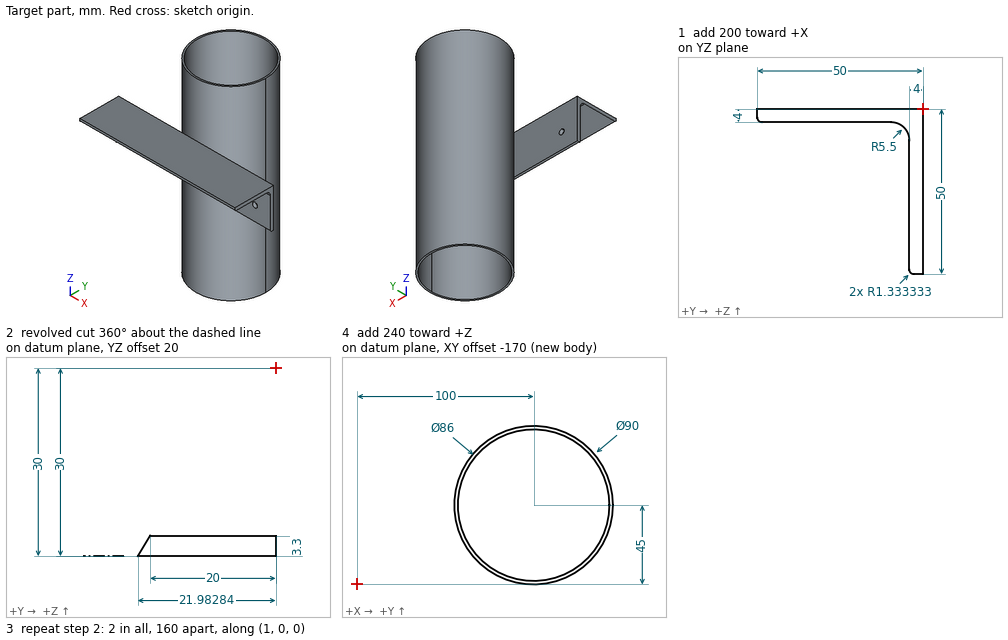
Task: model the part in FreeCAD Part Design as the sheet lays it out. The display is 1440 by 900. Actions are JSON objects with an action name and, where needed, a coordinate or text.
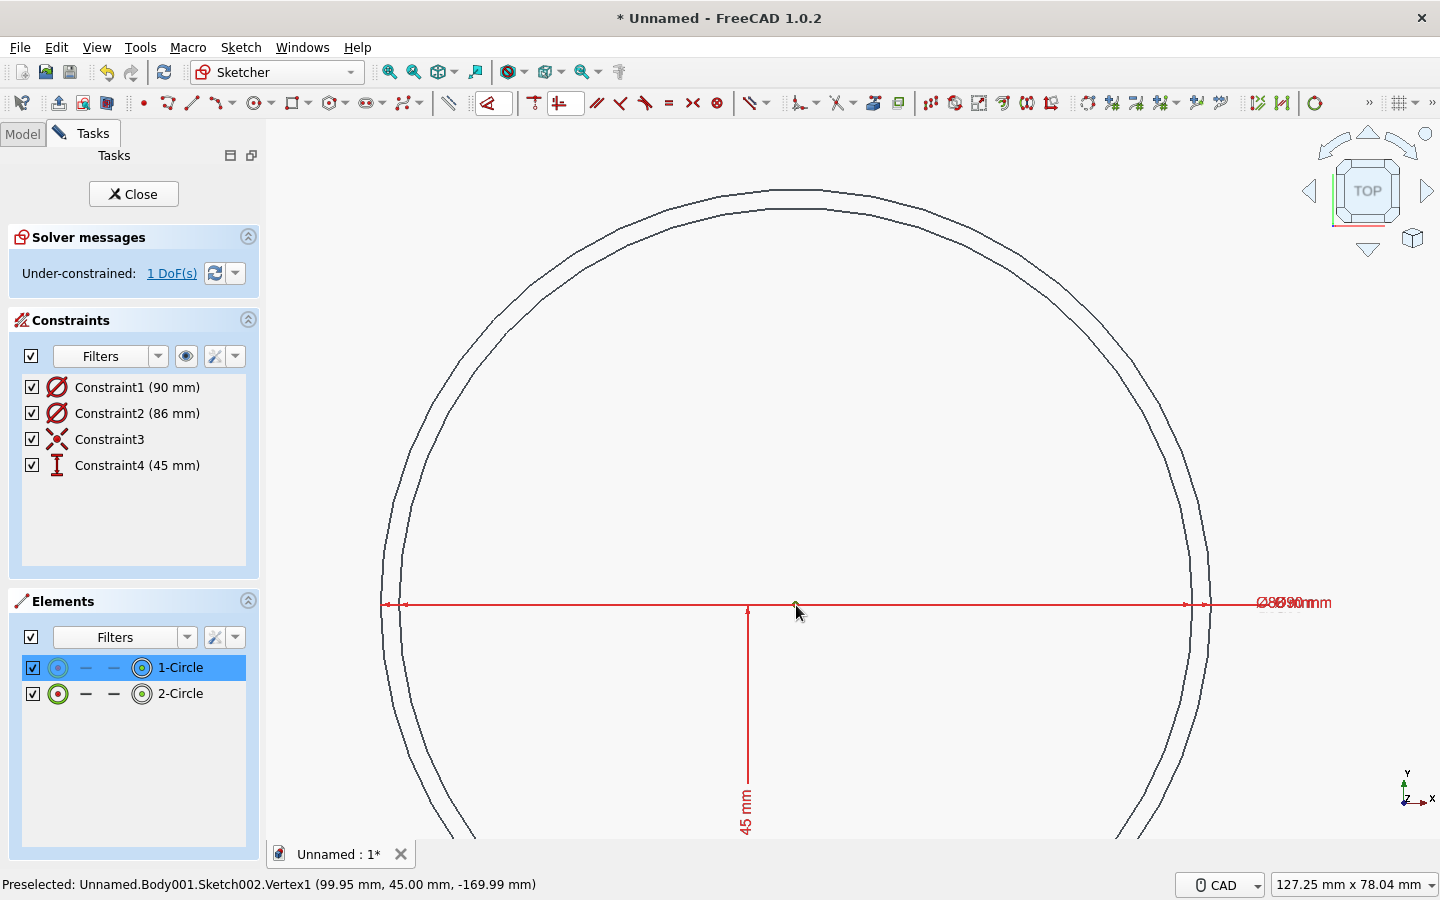
{"action": "left_click", "coordinate": [506, 104]}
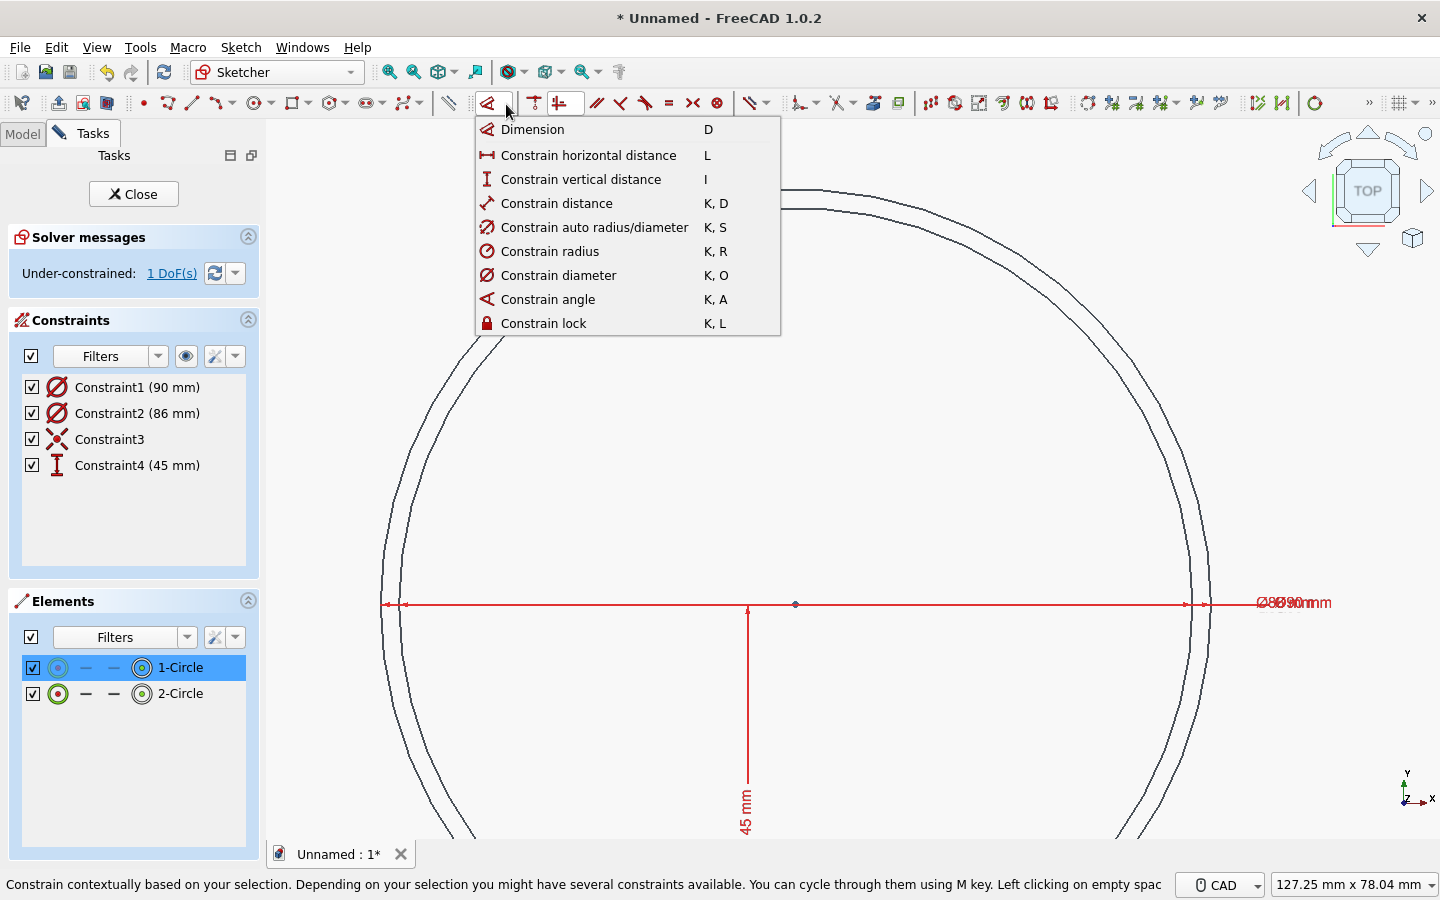
{"action": "left_click", "coordinate": [628, 155]}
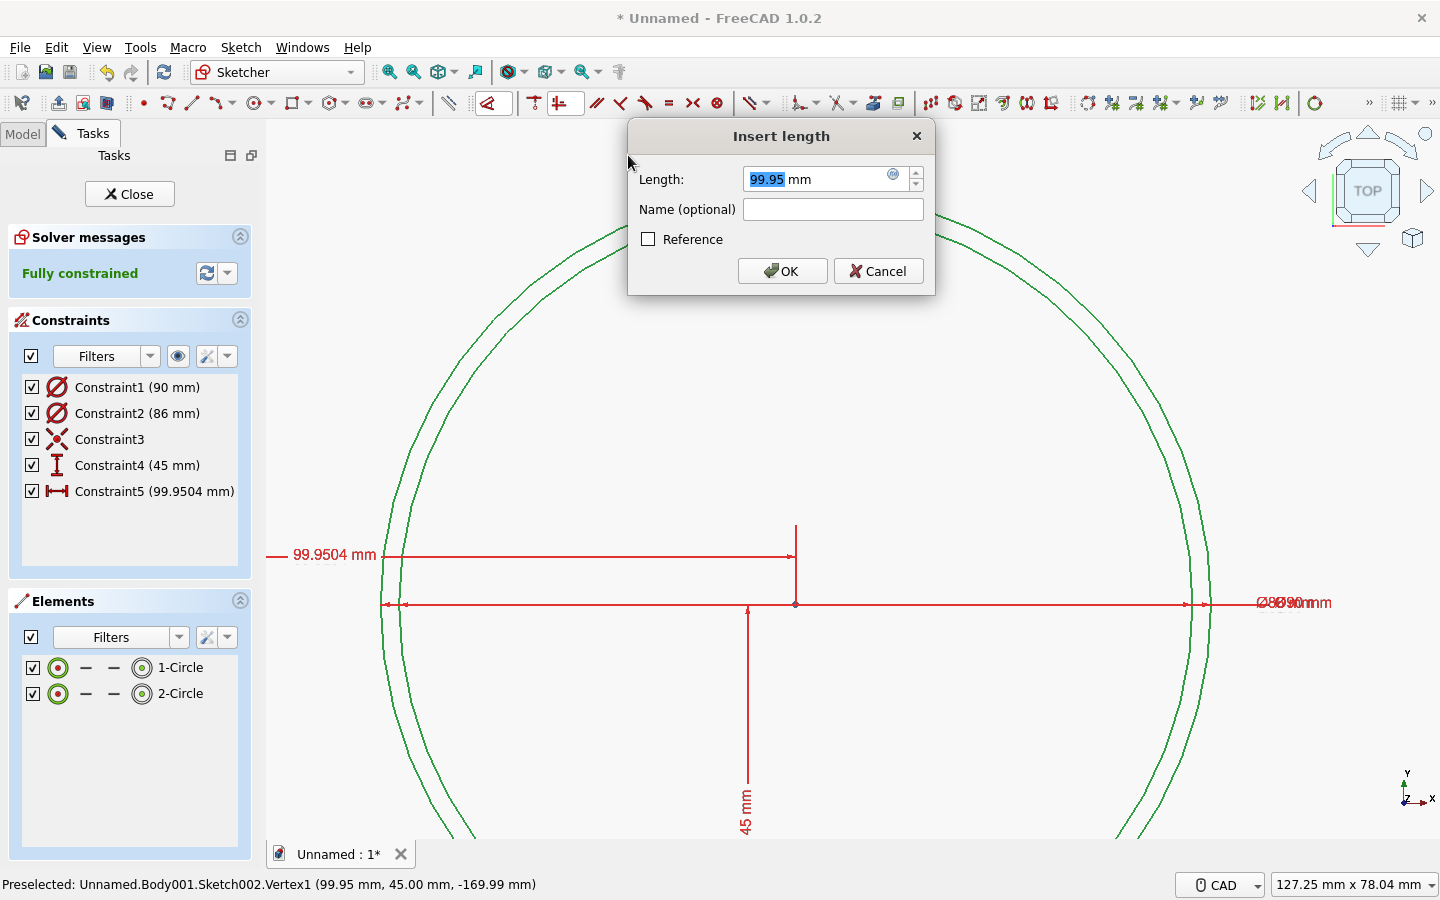
{"action": "type", "text": "100"}
{"action": "key", "text": "Return"}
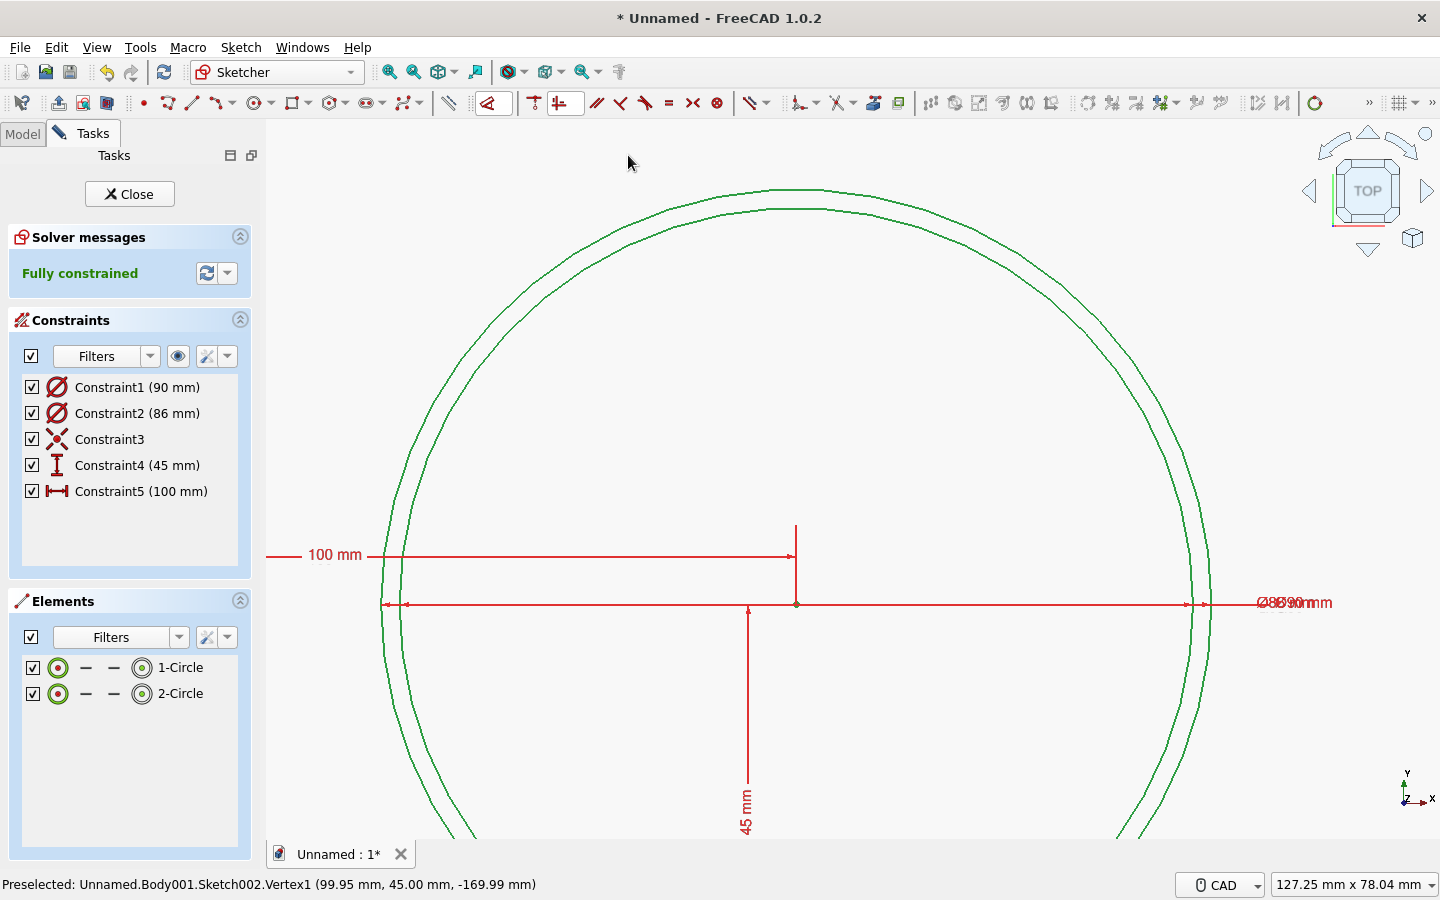
{"action": "left_click", "coordinate": [130, 194]}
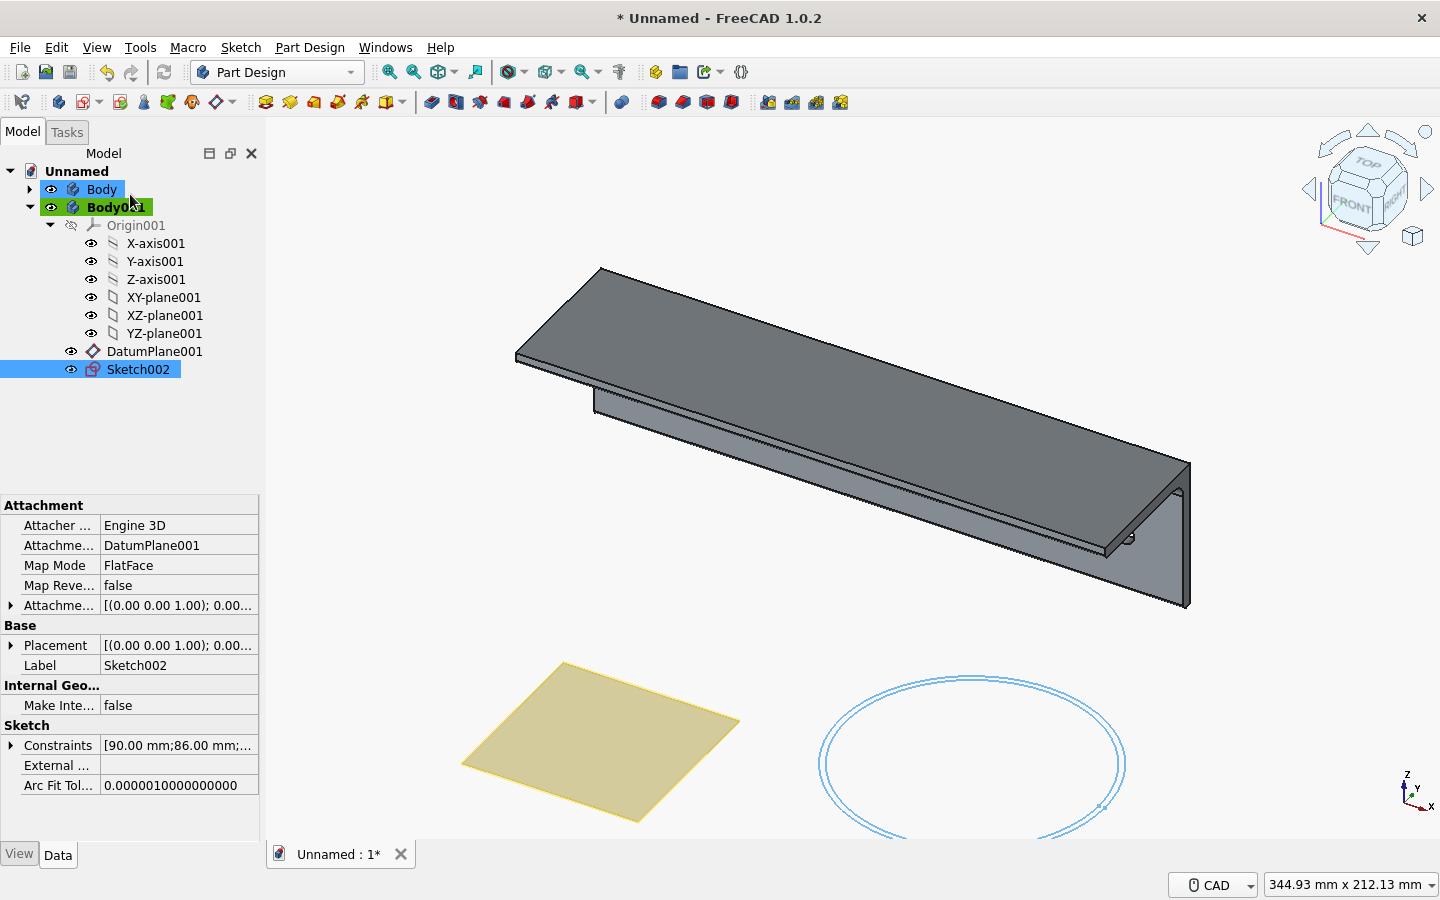
{"action": "left_click", "coordinate": [266, 102]}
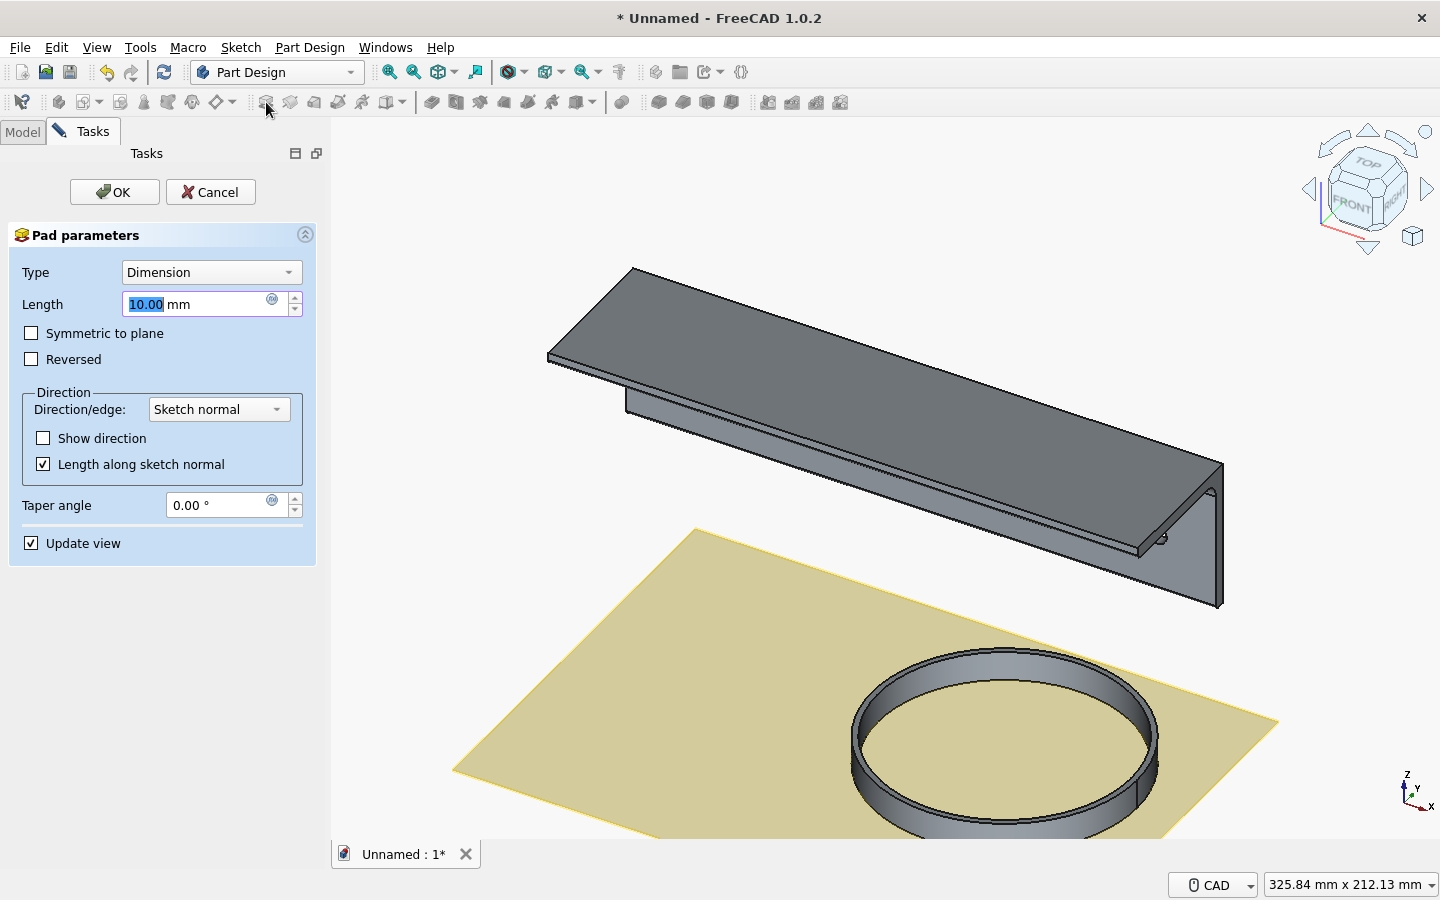
{"action": "type", "text": "240"}
{"action": "key", "text": "Tab"}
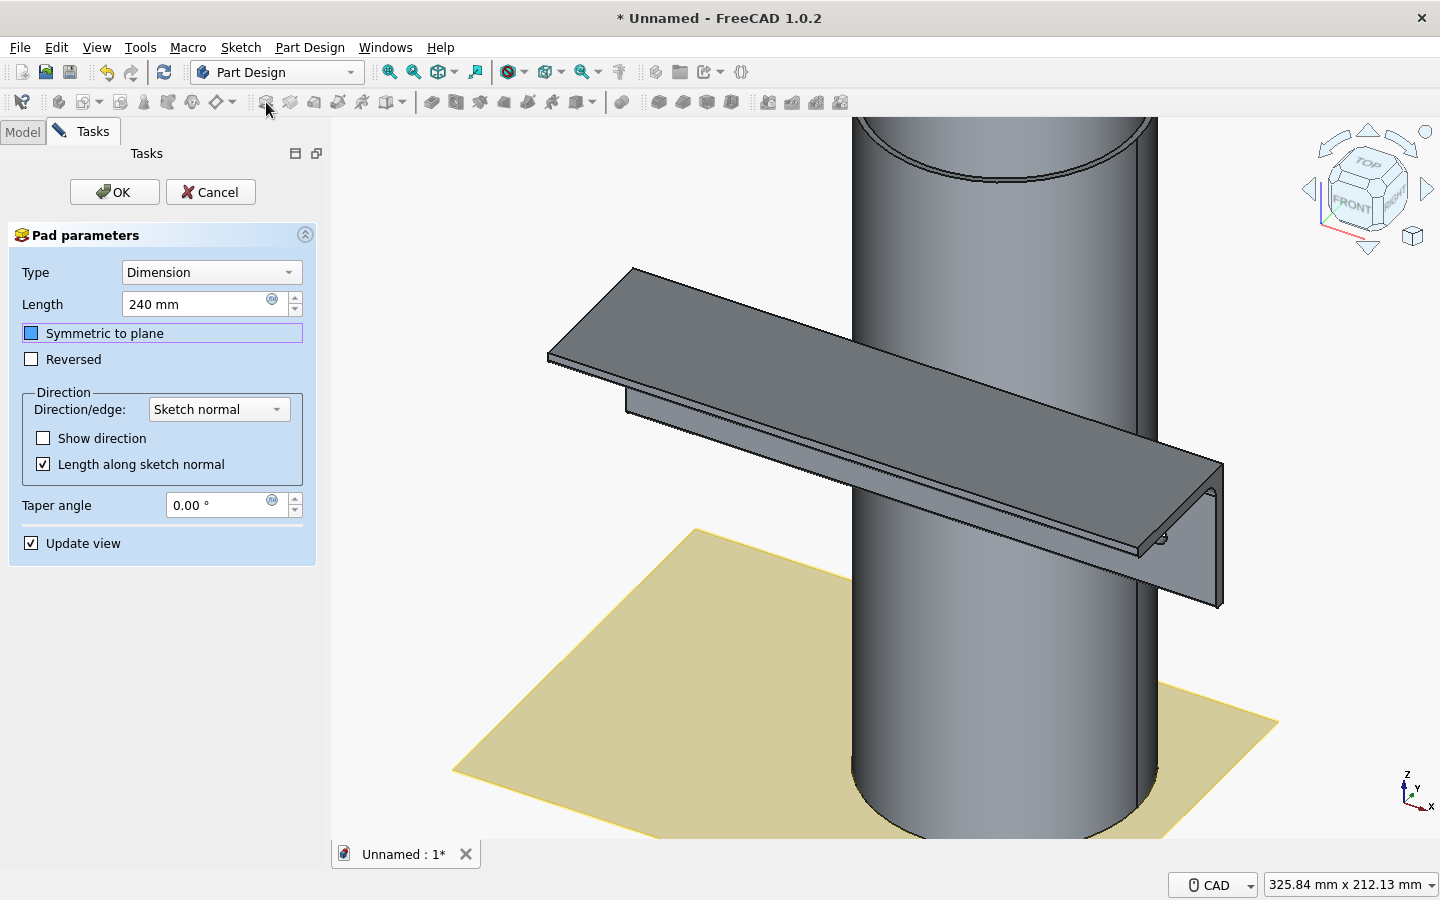
{"action": "left_click", "coordinate": [115, 192]}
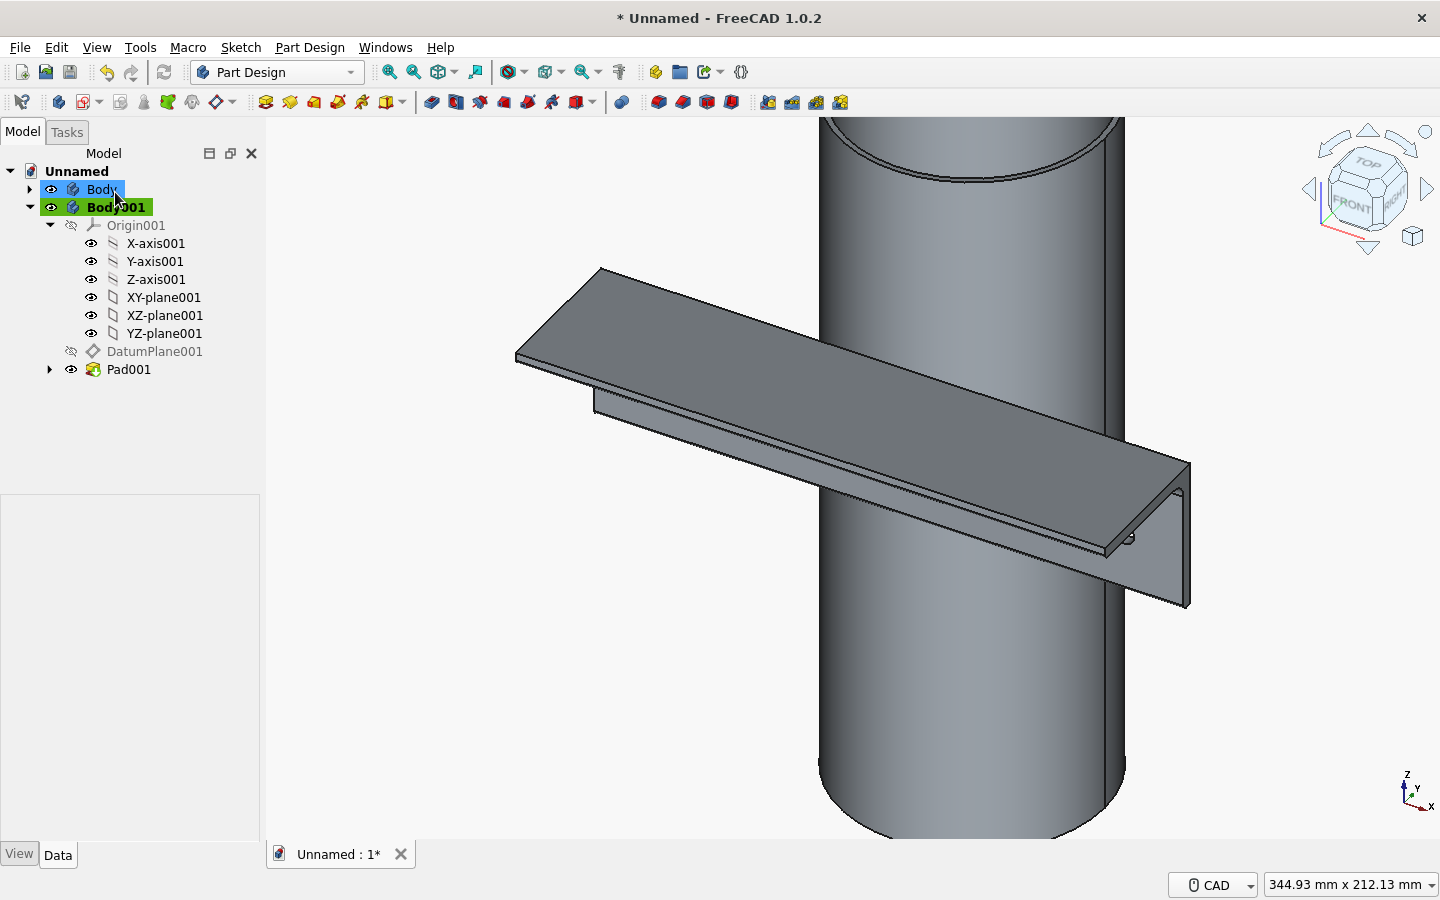
{"action": "key", "text": "0"}